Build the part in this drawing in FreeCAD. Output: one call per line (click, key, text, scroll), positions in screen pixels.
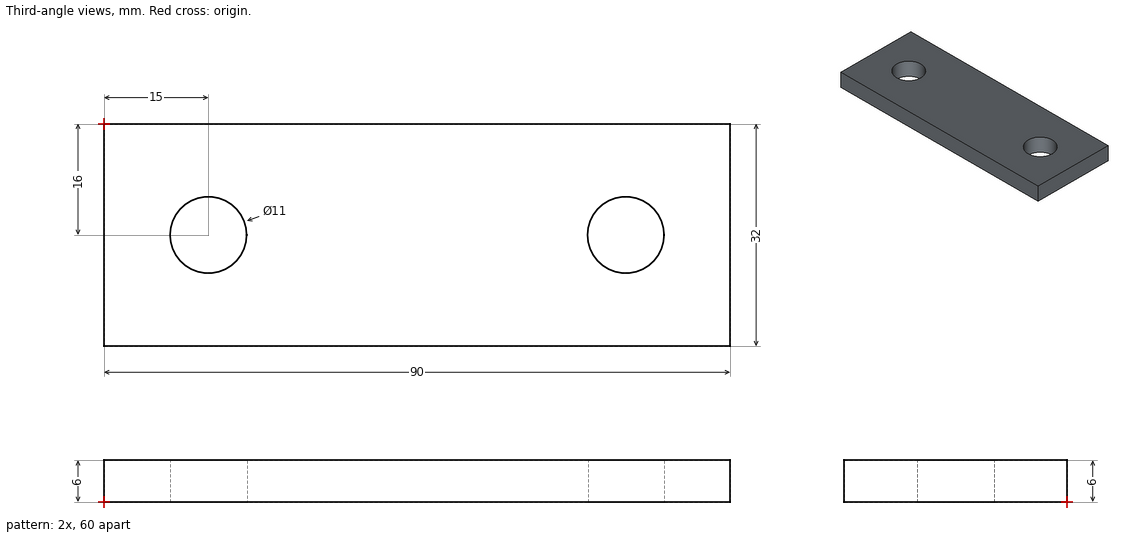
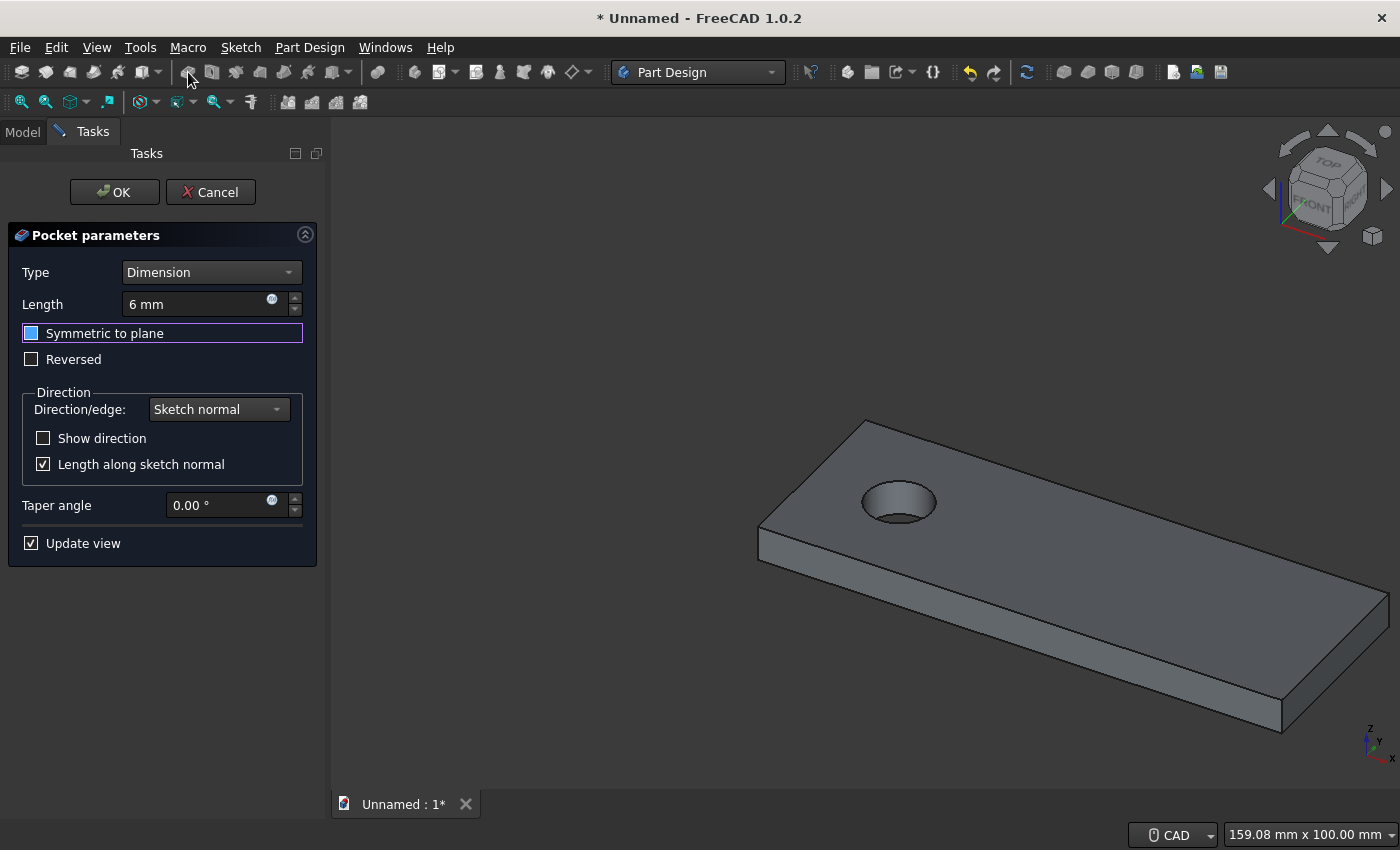
click(115, 192)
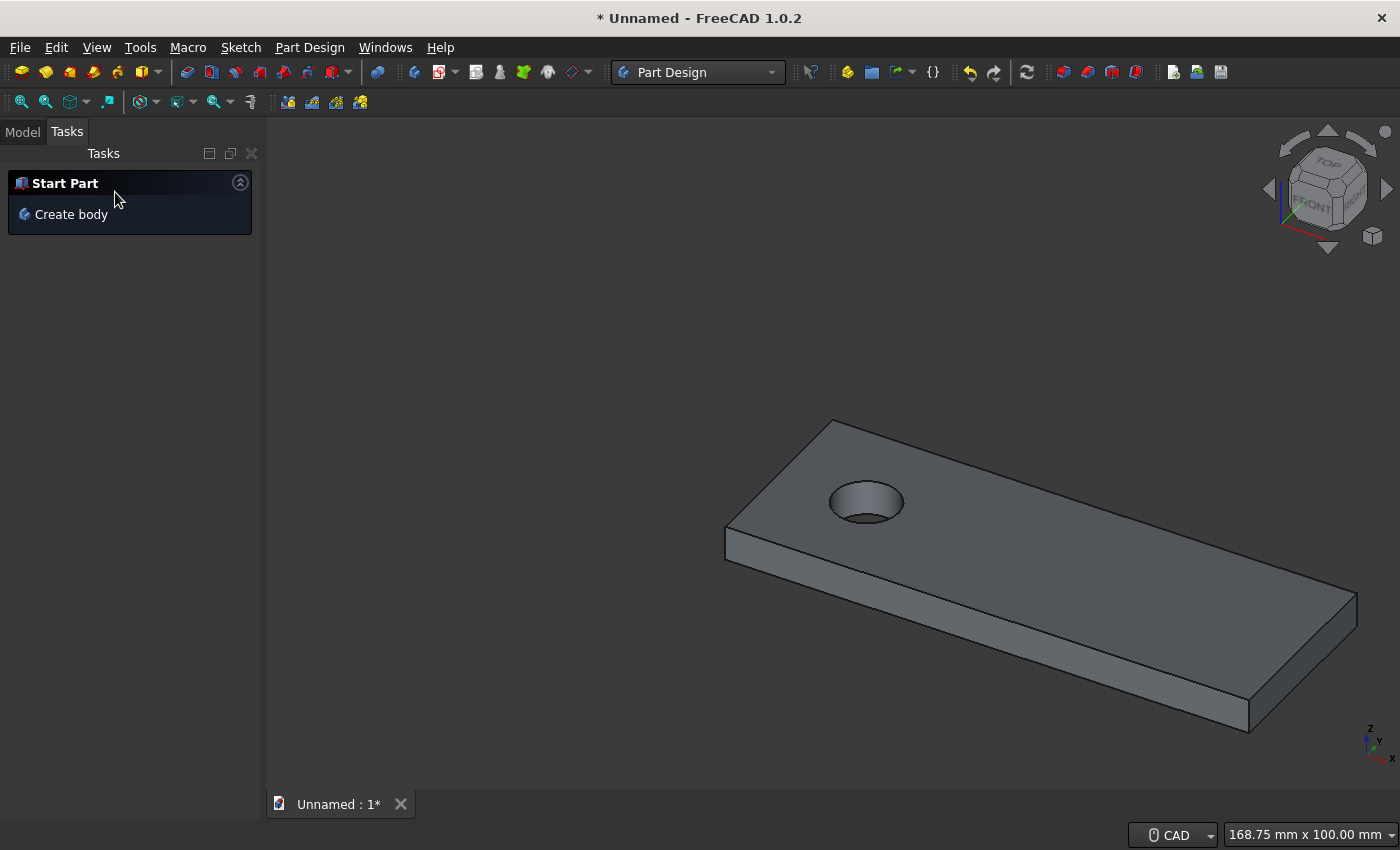
click(23, 131)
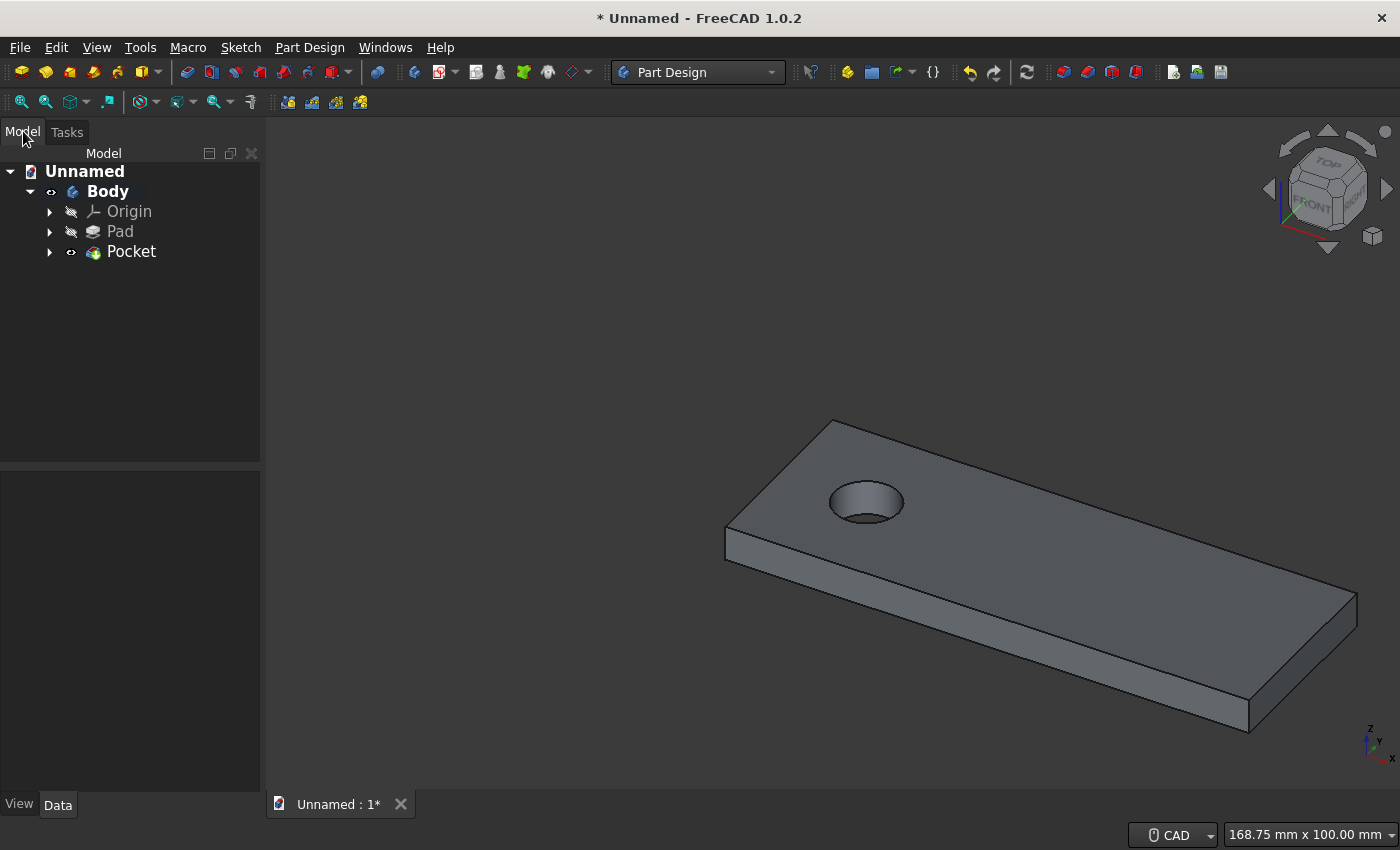
click(116, 252)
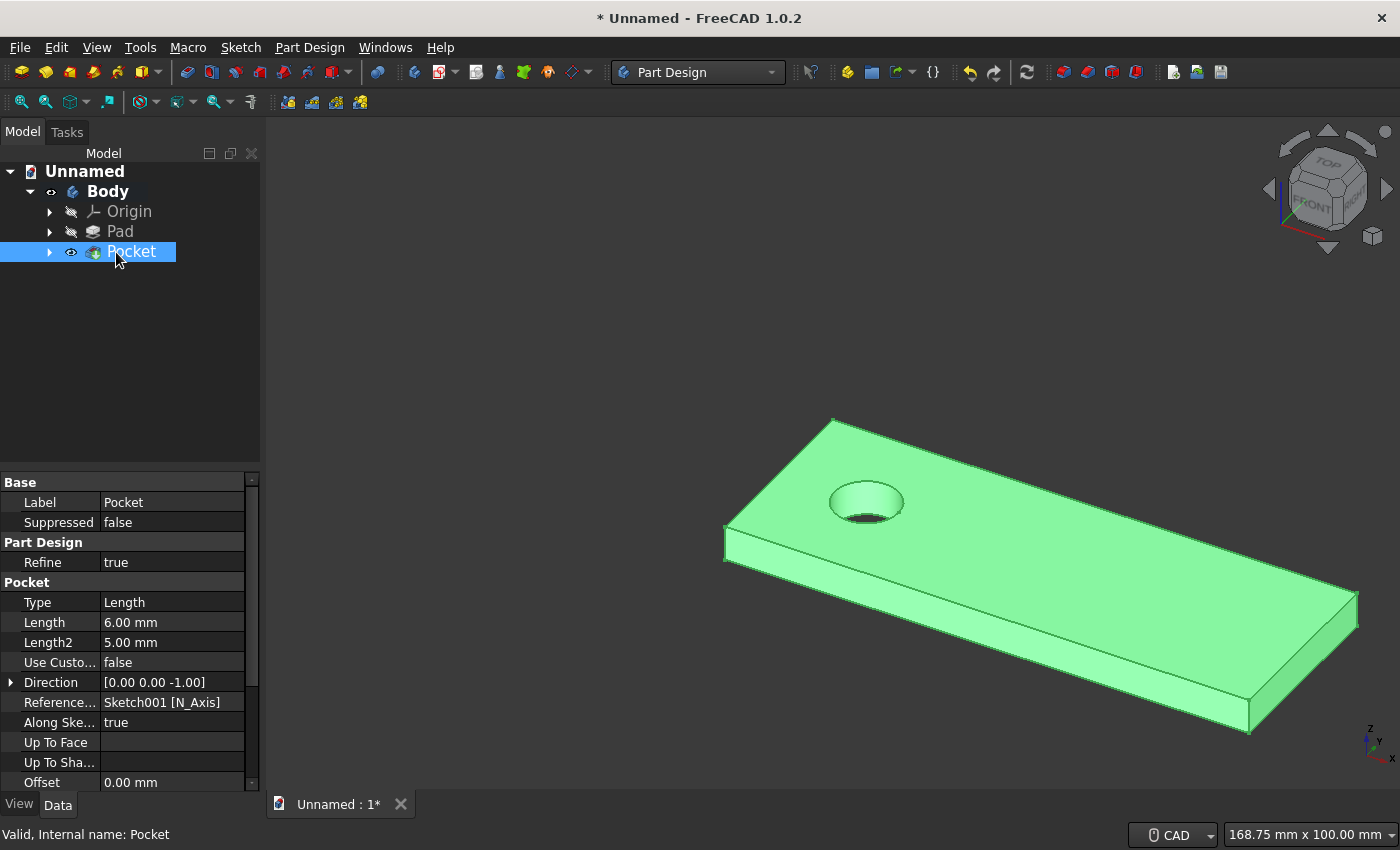
click(312, 102)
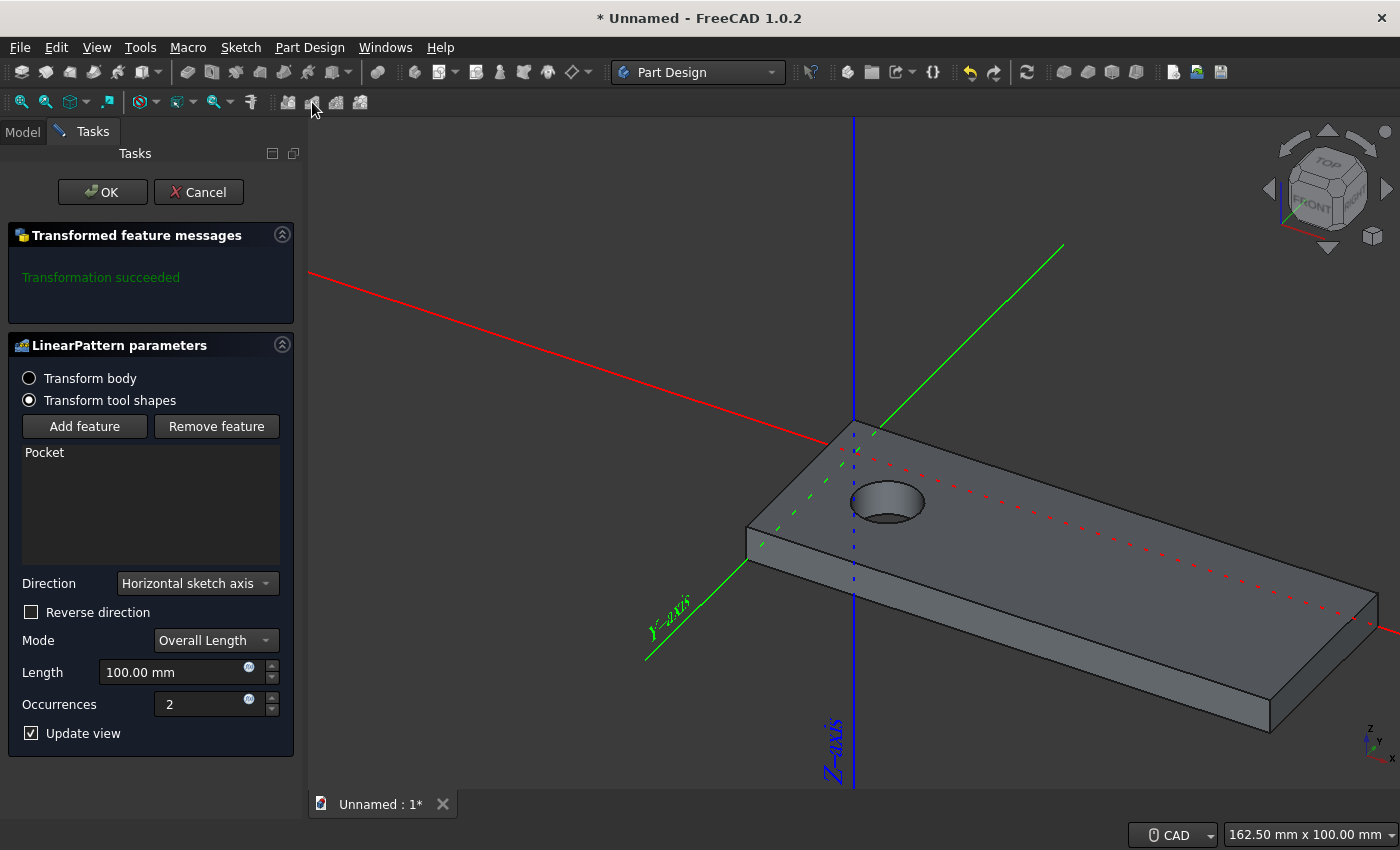
click(198, 584)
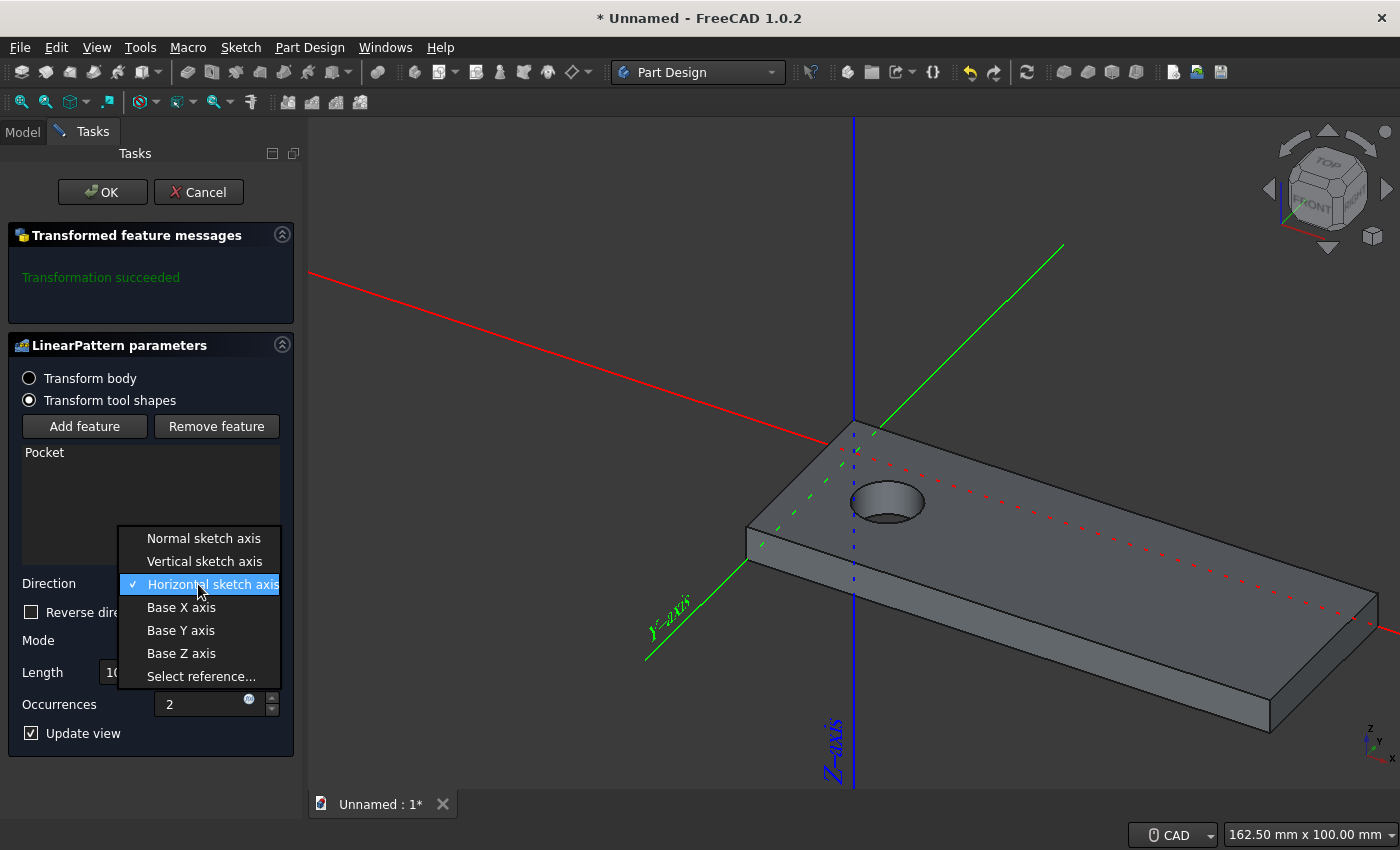
click(198, 608)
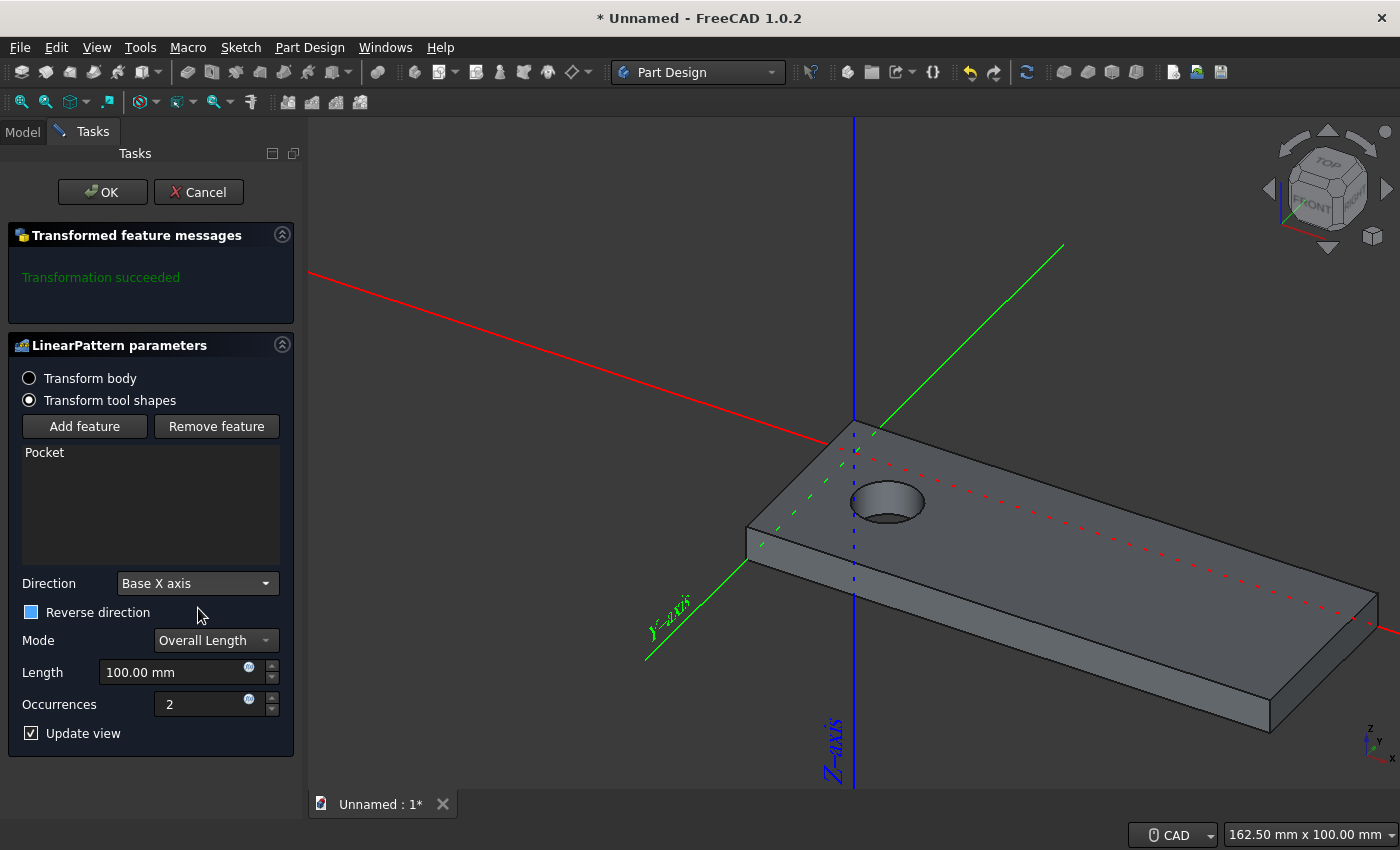
click(217, 640)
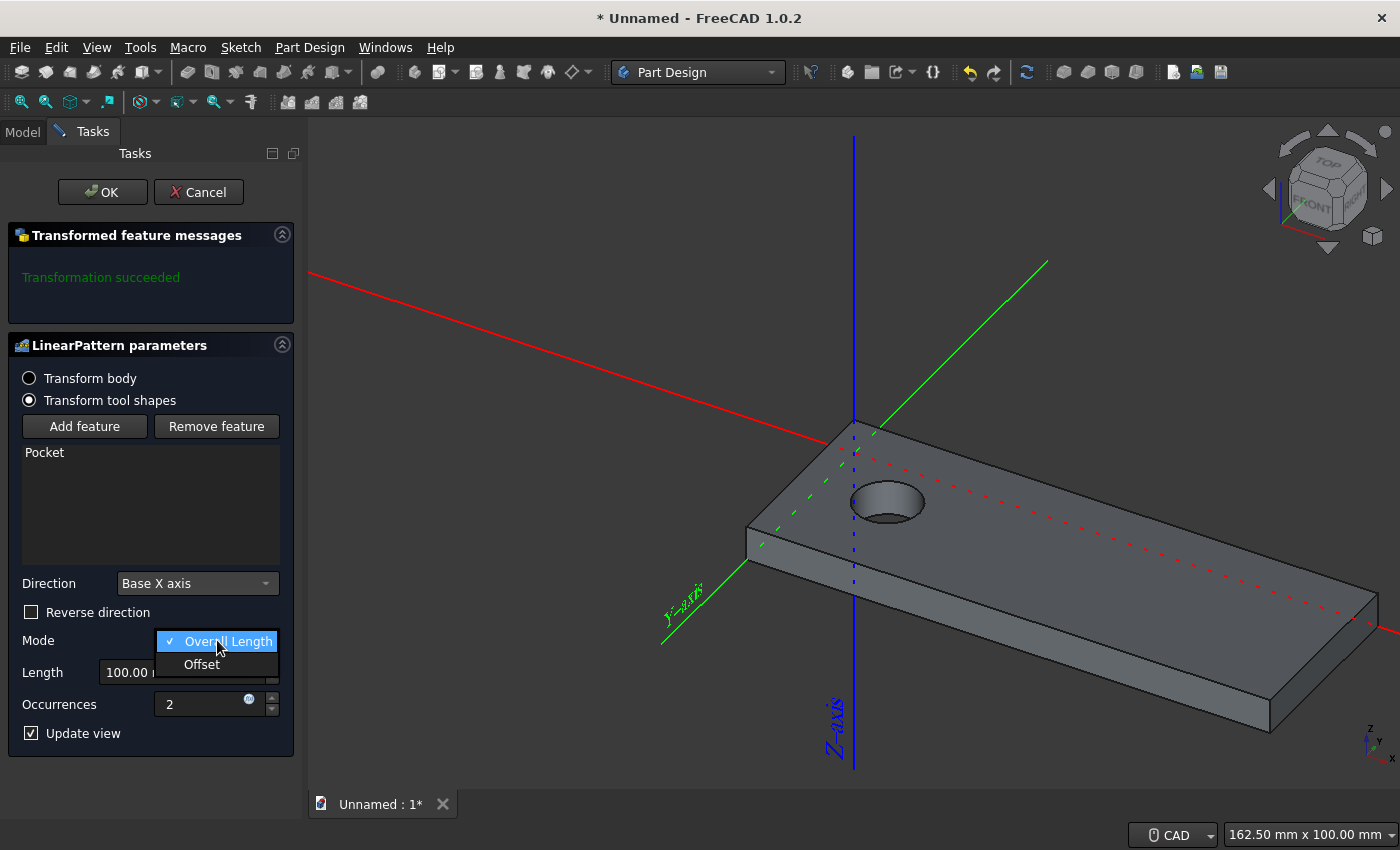
click(216, 664)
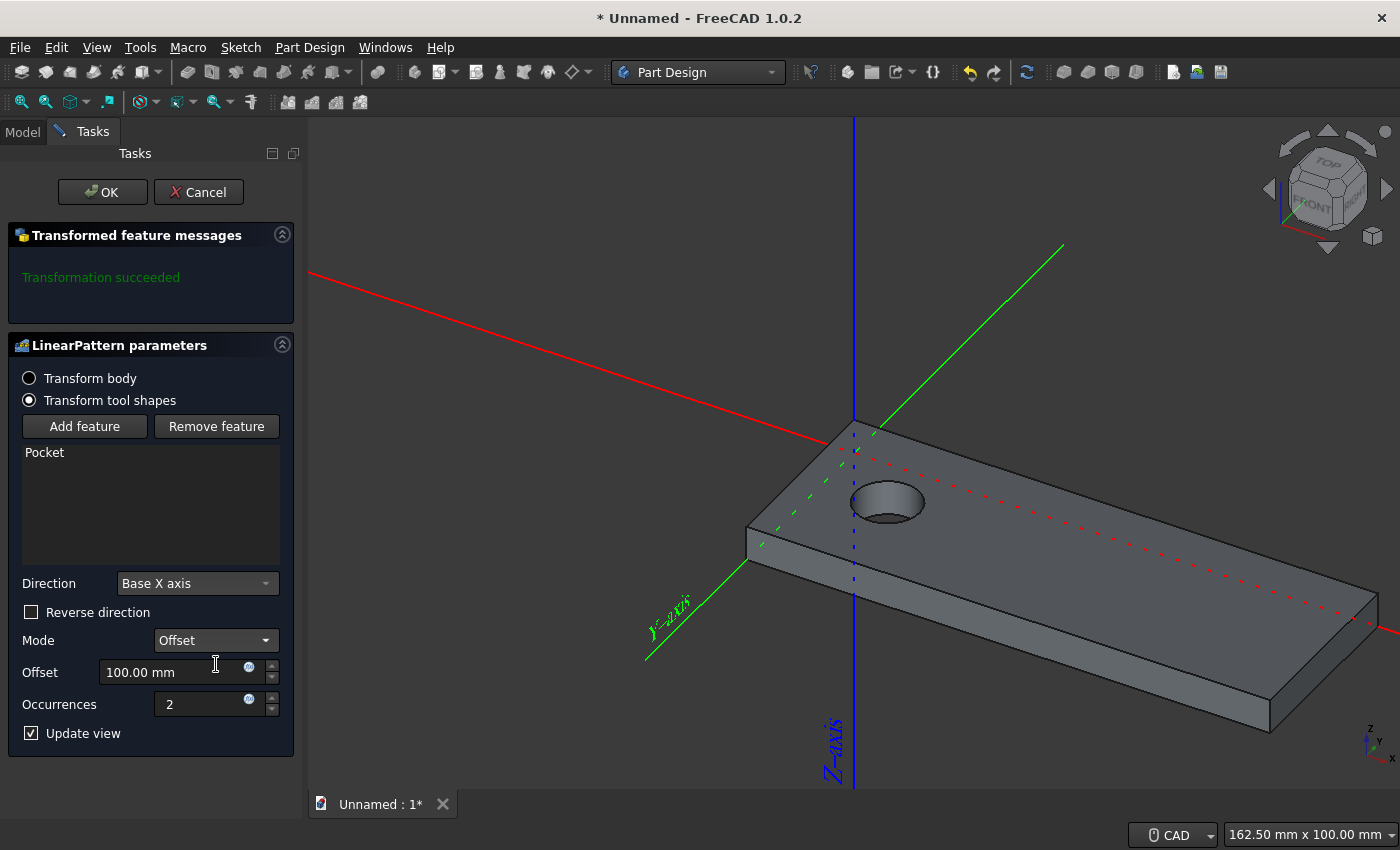
triple_click(182, 672)